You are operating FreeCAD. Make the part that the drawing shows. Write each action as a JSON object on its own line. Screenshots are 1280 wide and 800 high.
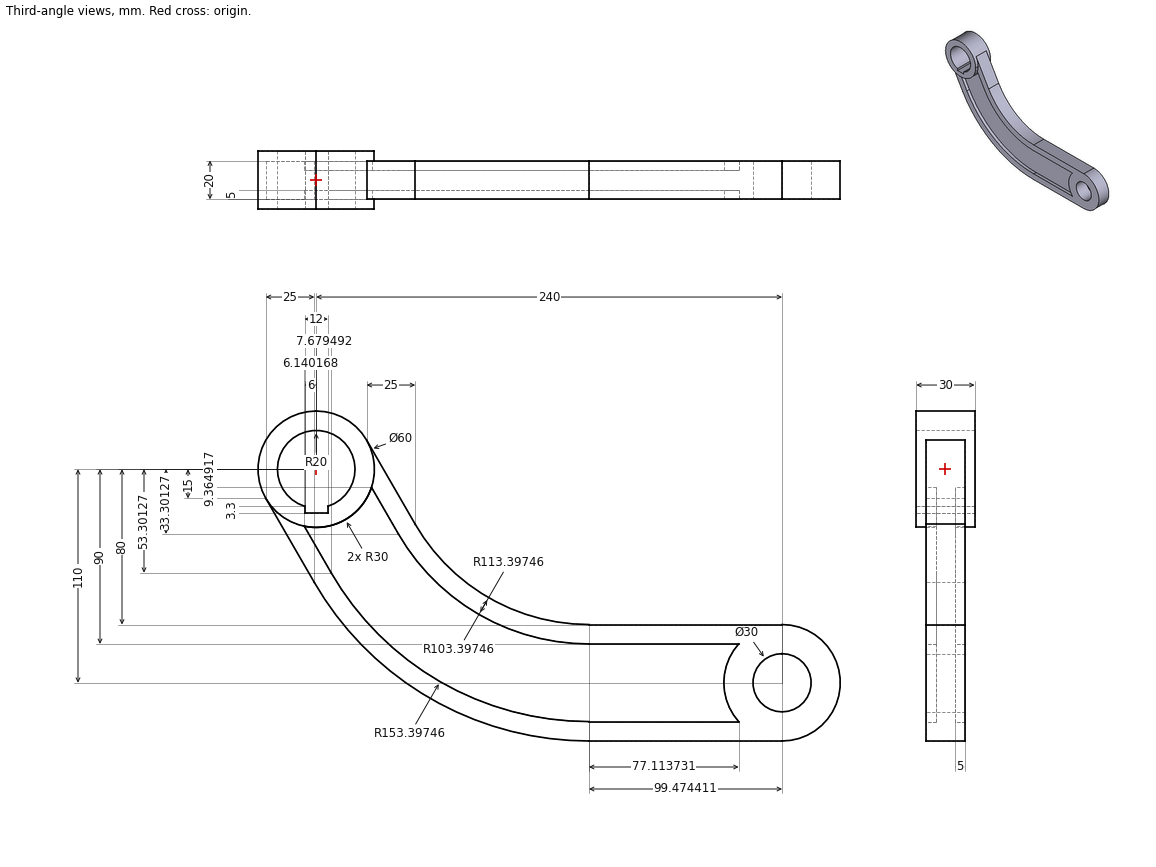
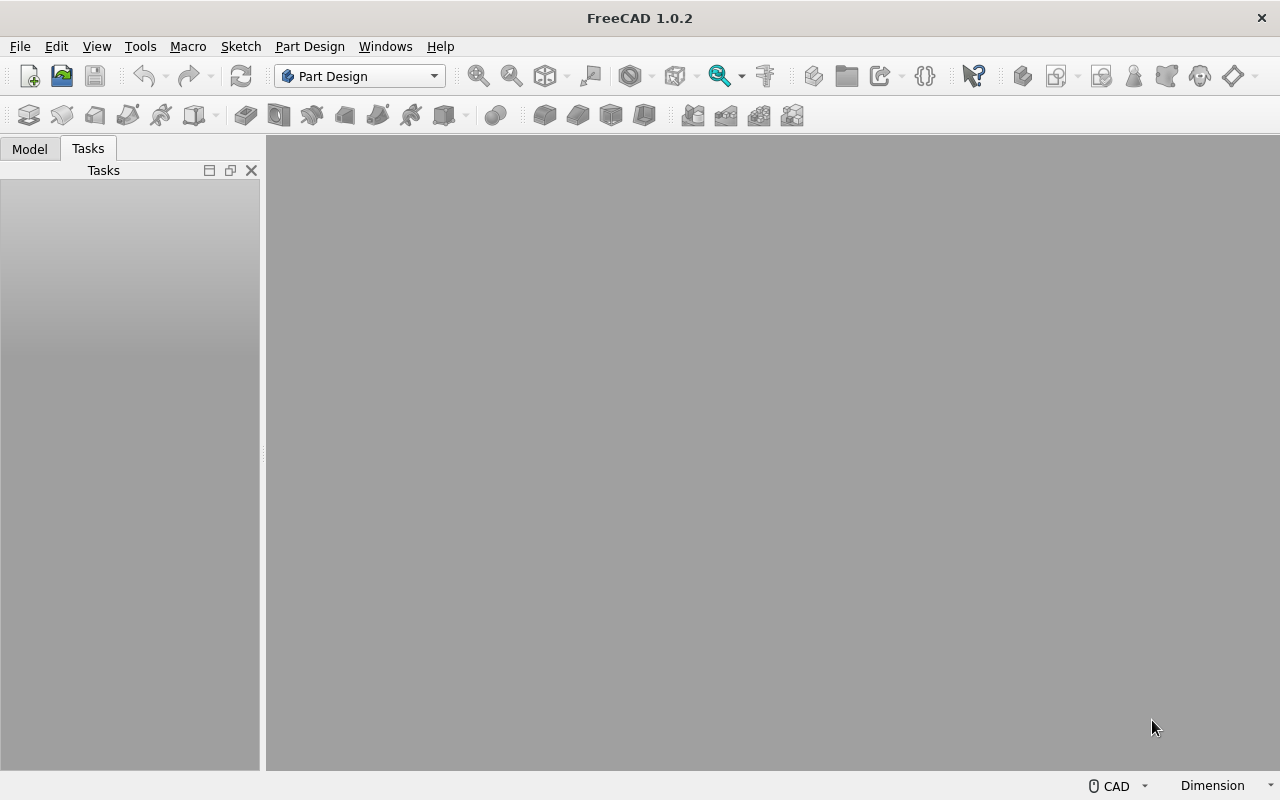
{"action": "left_click", "coordinate": [29, 76]}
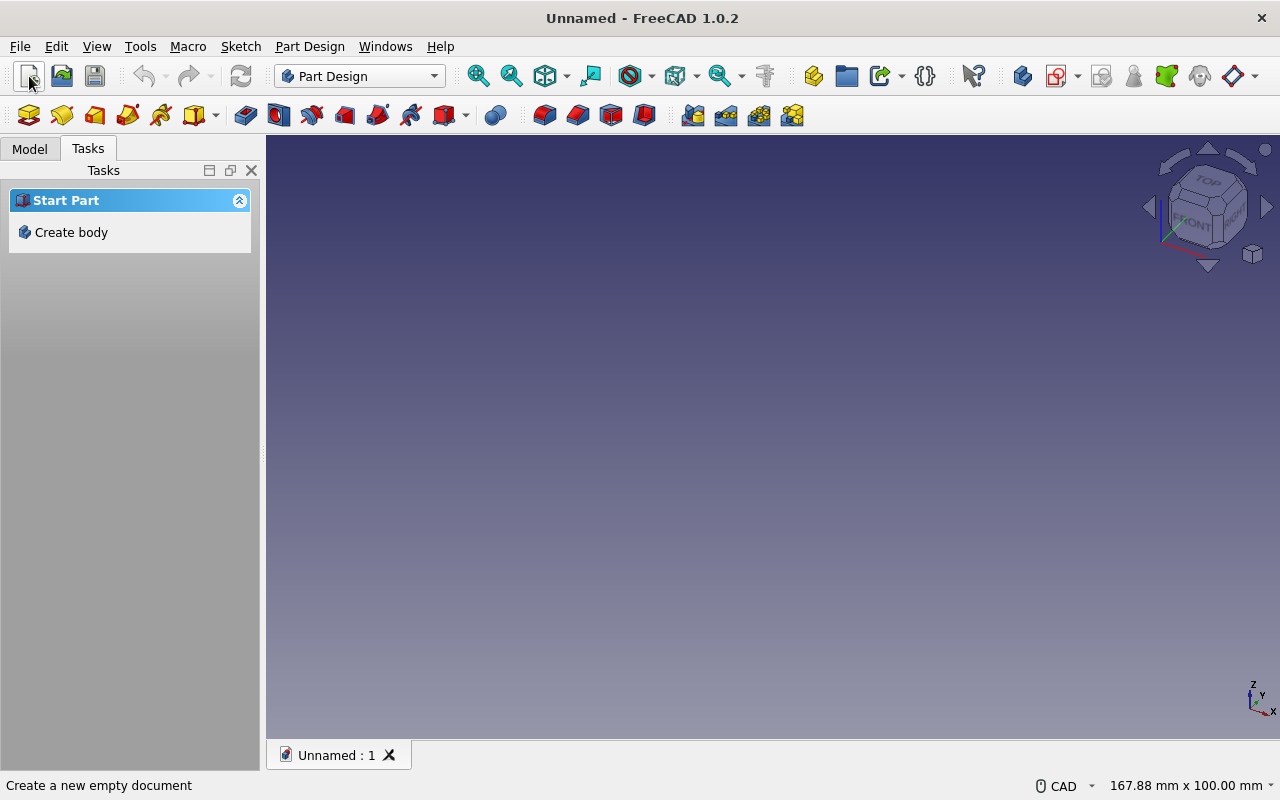
{"action": "left_click", "coordinate": [1056, 76]}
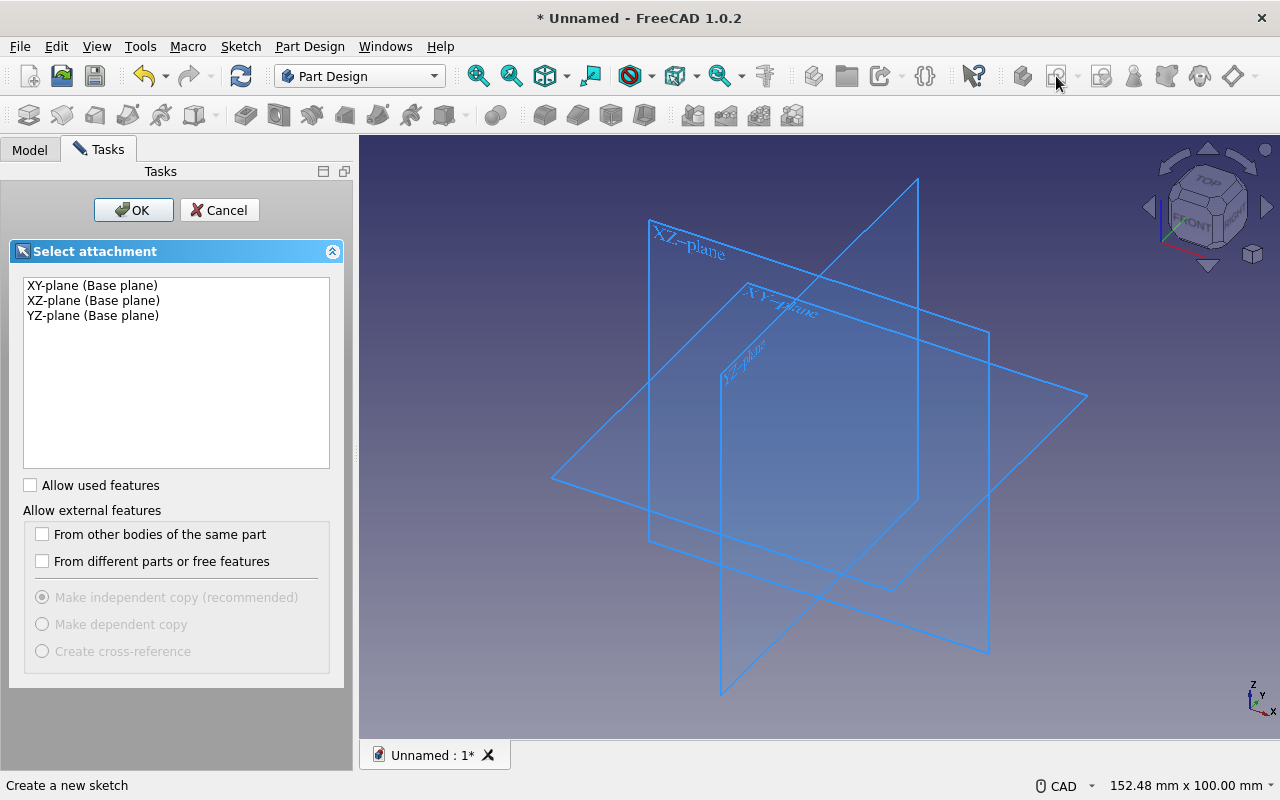
{"action": "left_click", "coordinate": [84, 300]}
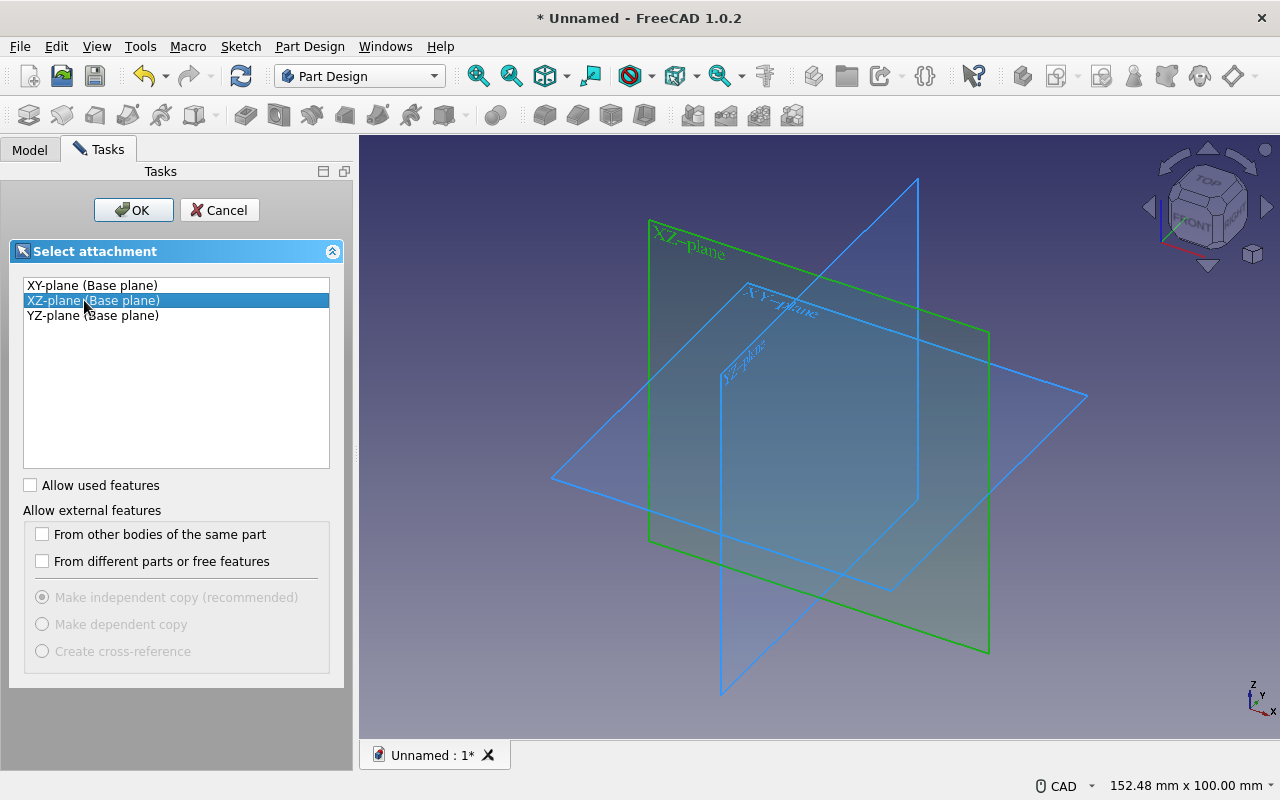
{"action": "left_click", "coordinate": [134, 210]}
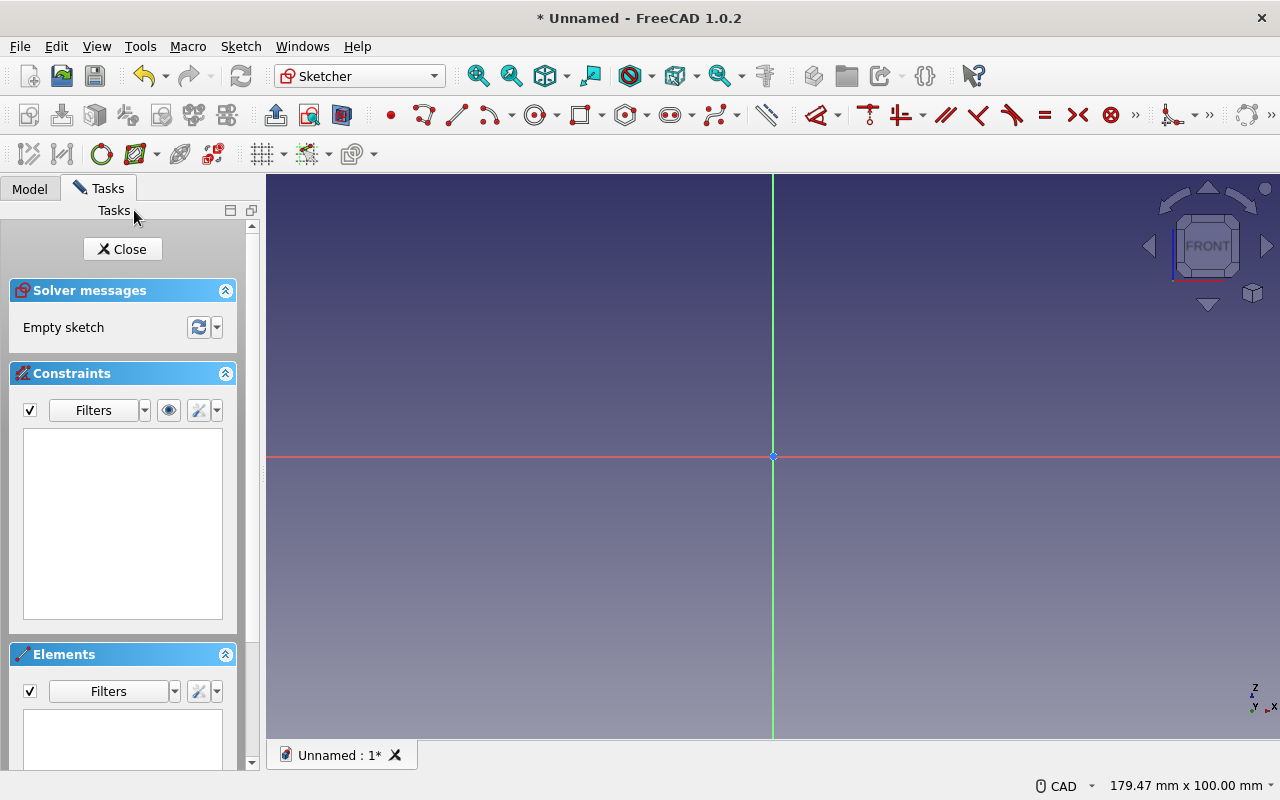
{"action": "left_click", "coordinate": [424, 116]}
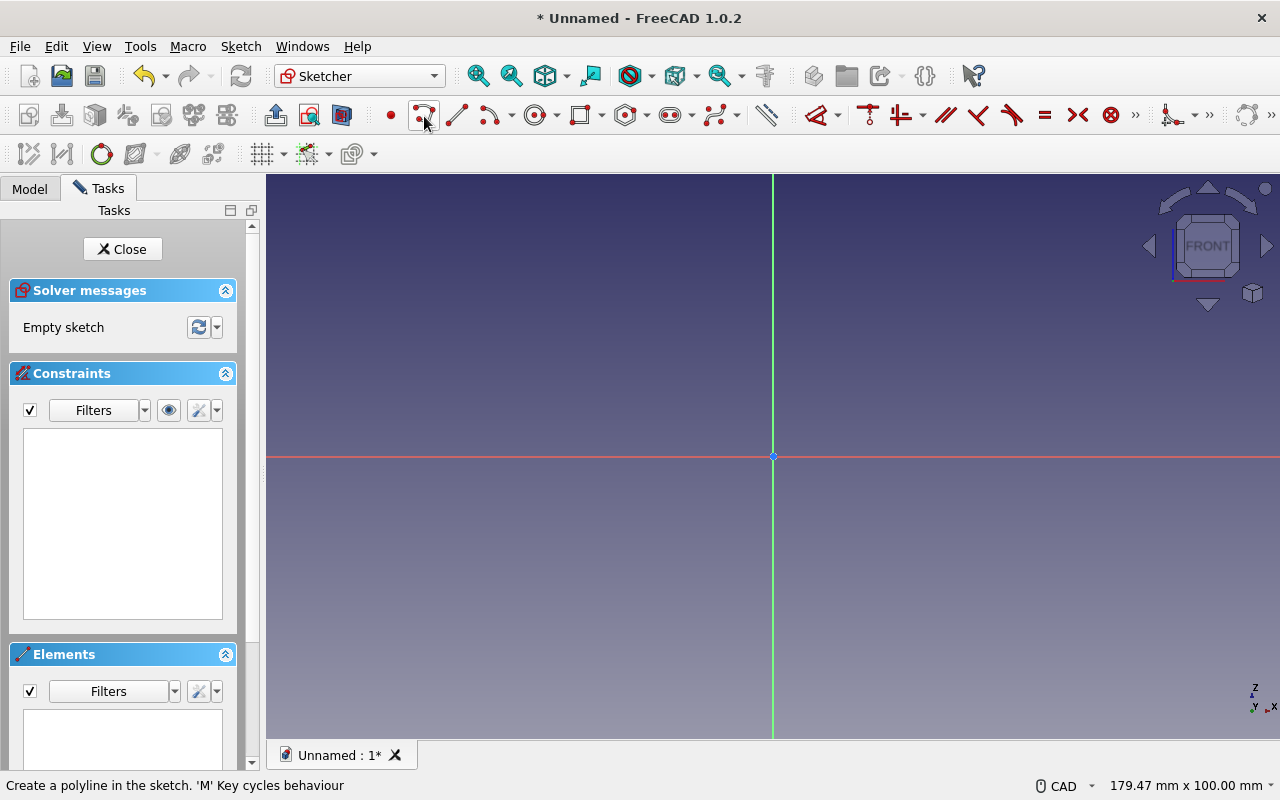
{"action": "left_click", "coordinate": [739, 564]}
{"action": "left_click", "coordinate": [739, 583]}
{"action": "left_click", "coordinate": [807, 583]}
{"action": "left_click", "coordinate": [807, 564]}
{"action": "right_click", "coordinate": [807, 564]}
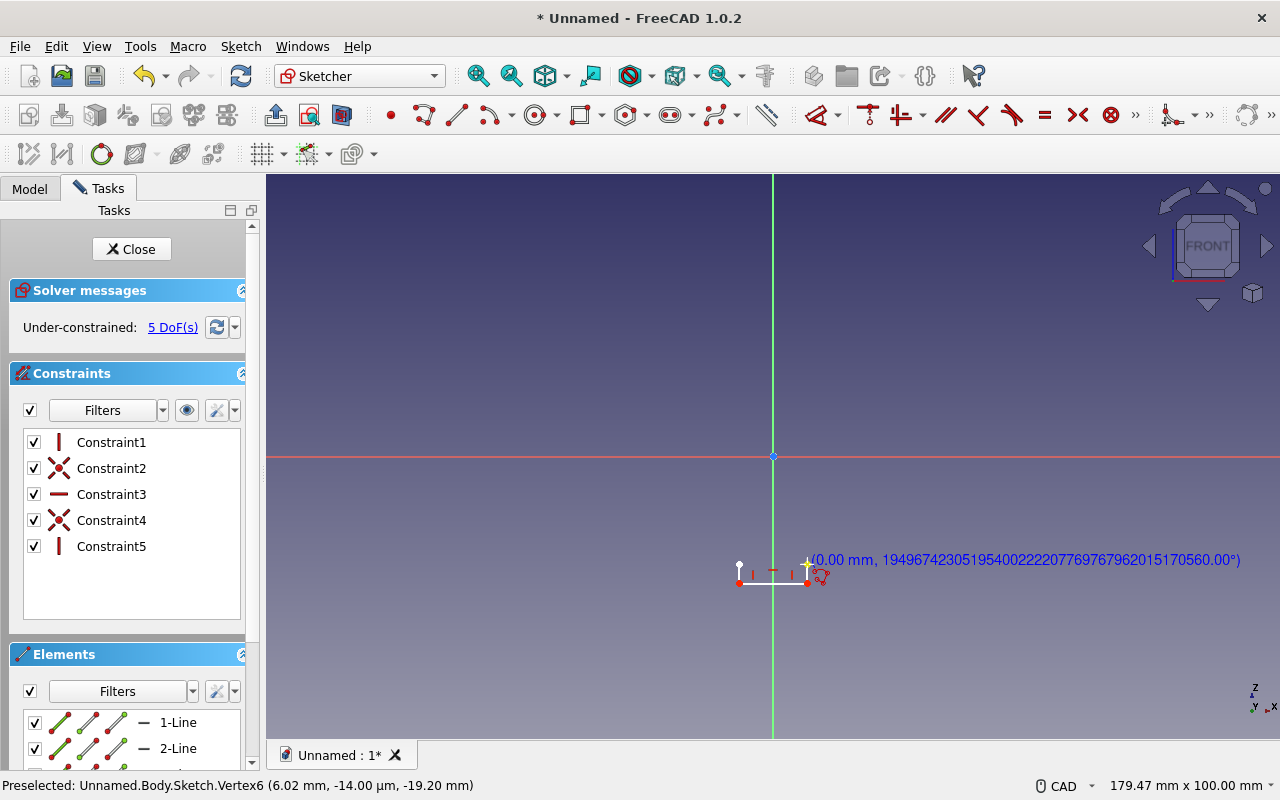
{"action": "left_click", "coordinate": [512, 116]}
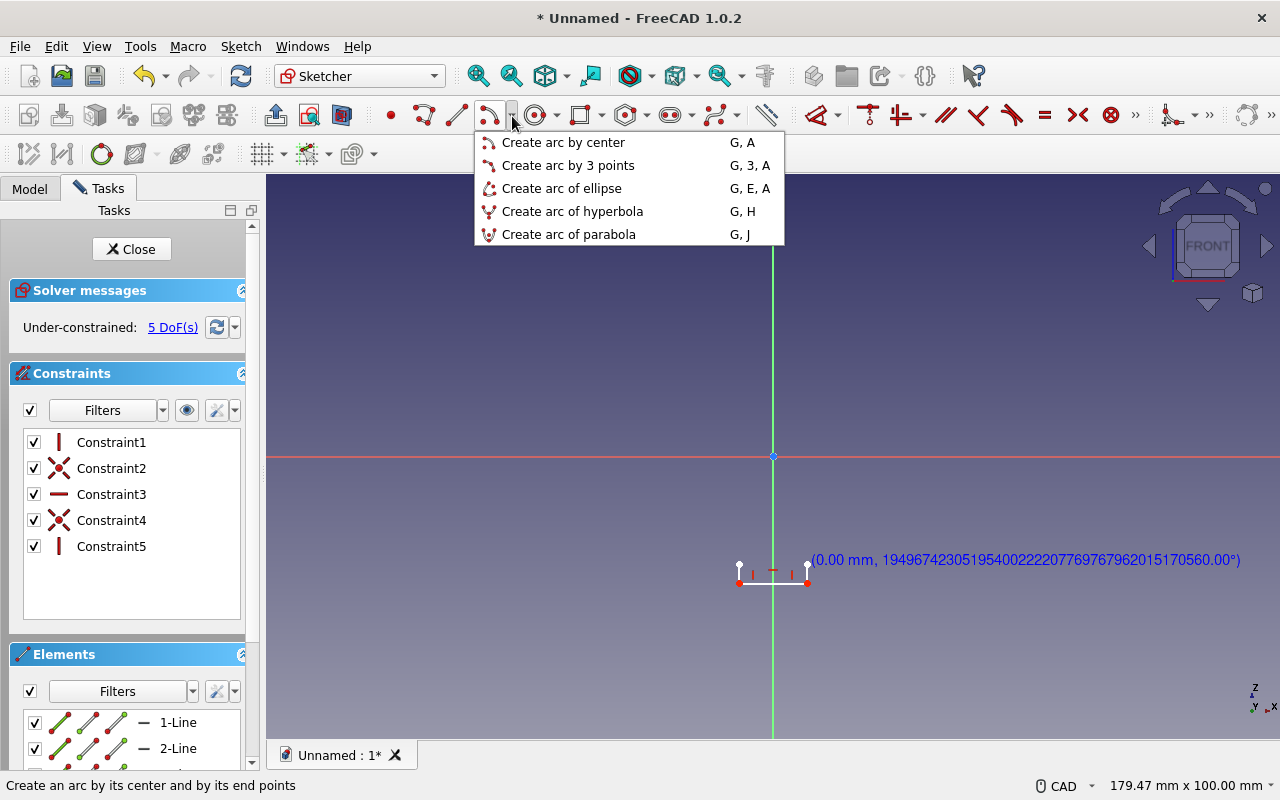
{"action": "left_click", "coordinate": [630, 166]}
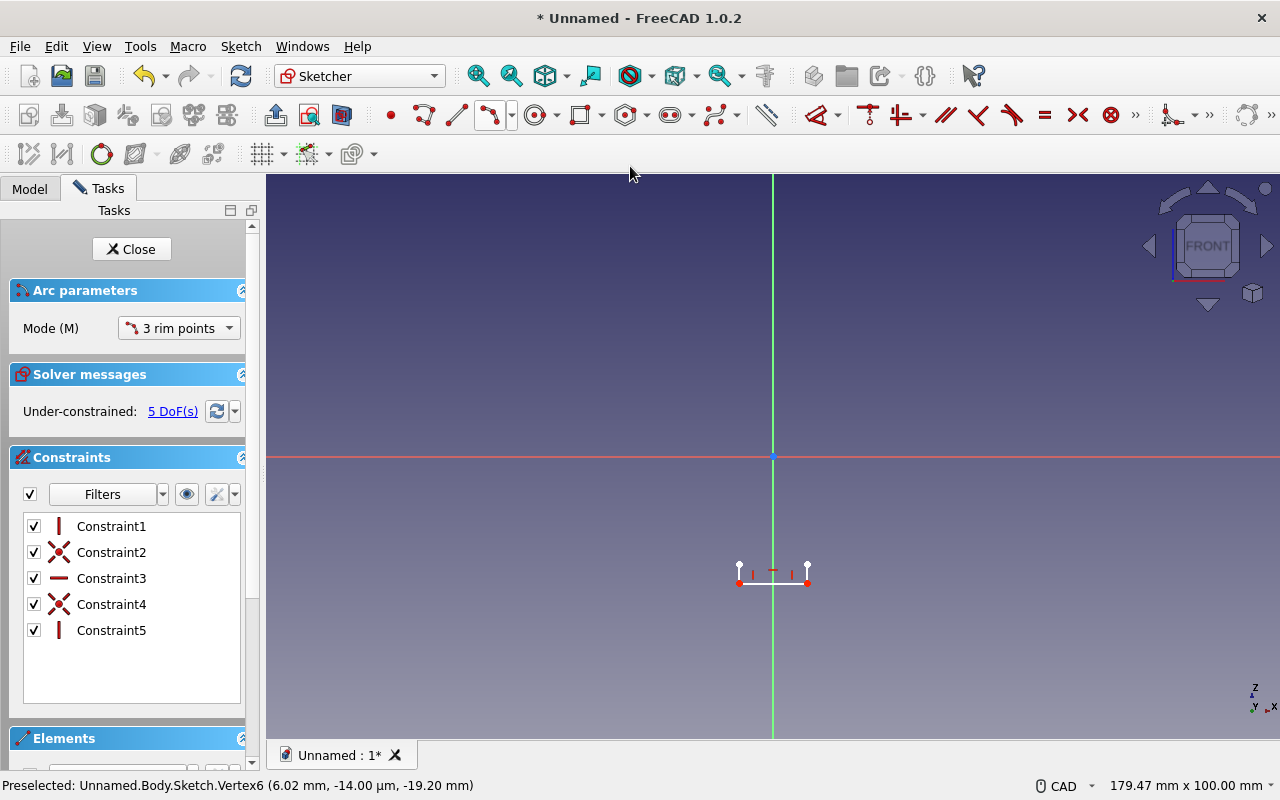
{"action": "scroll", "coordinate": [807, 564], "scroll_direction": "up", "scroll_amount": 3}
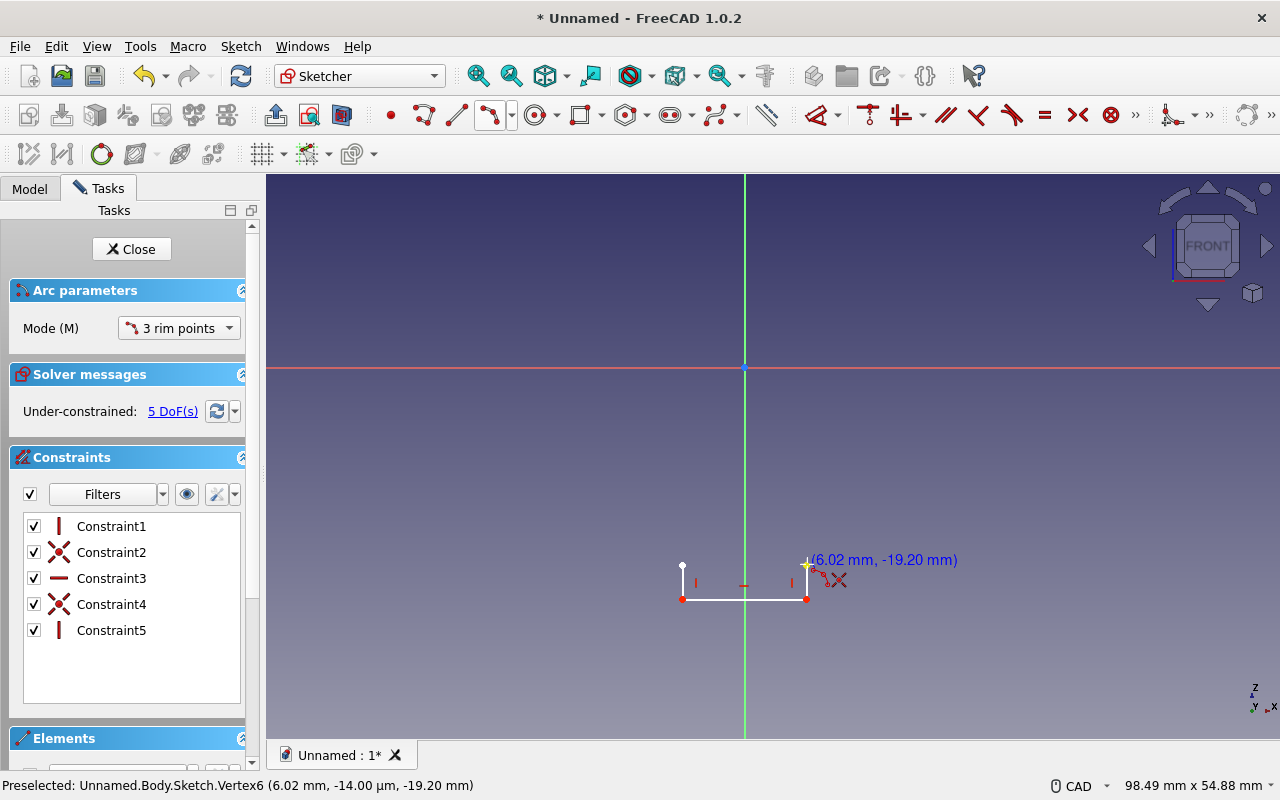
{"action": "left_click", "coordinate": [807, 565]}
{"action": "left_click", "coordinate": [683, 565]}